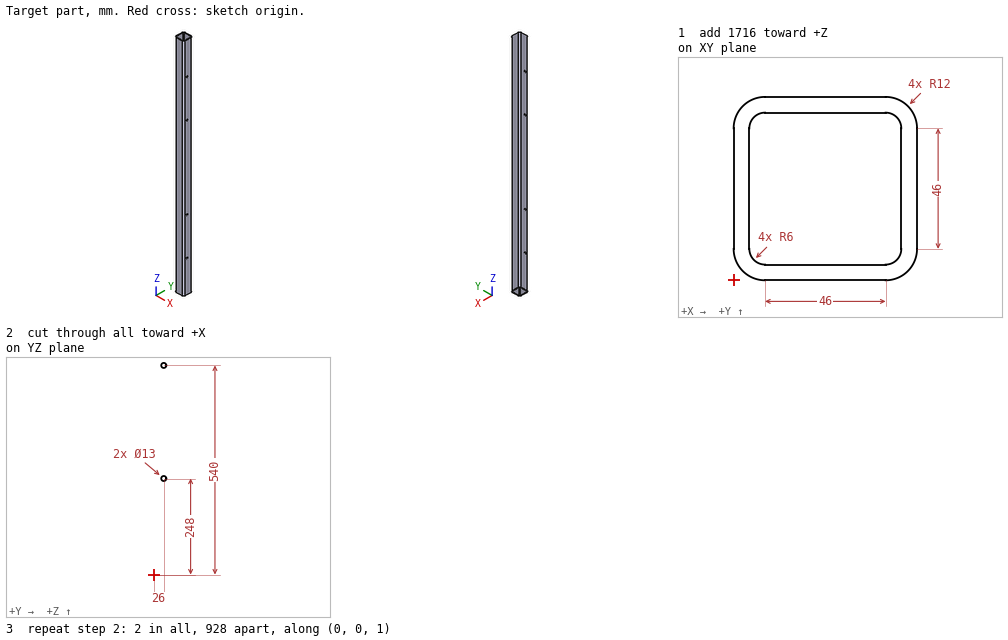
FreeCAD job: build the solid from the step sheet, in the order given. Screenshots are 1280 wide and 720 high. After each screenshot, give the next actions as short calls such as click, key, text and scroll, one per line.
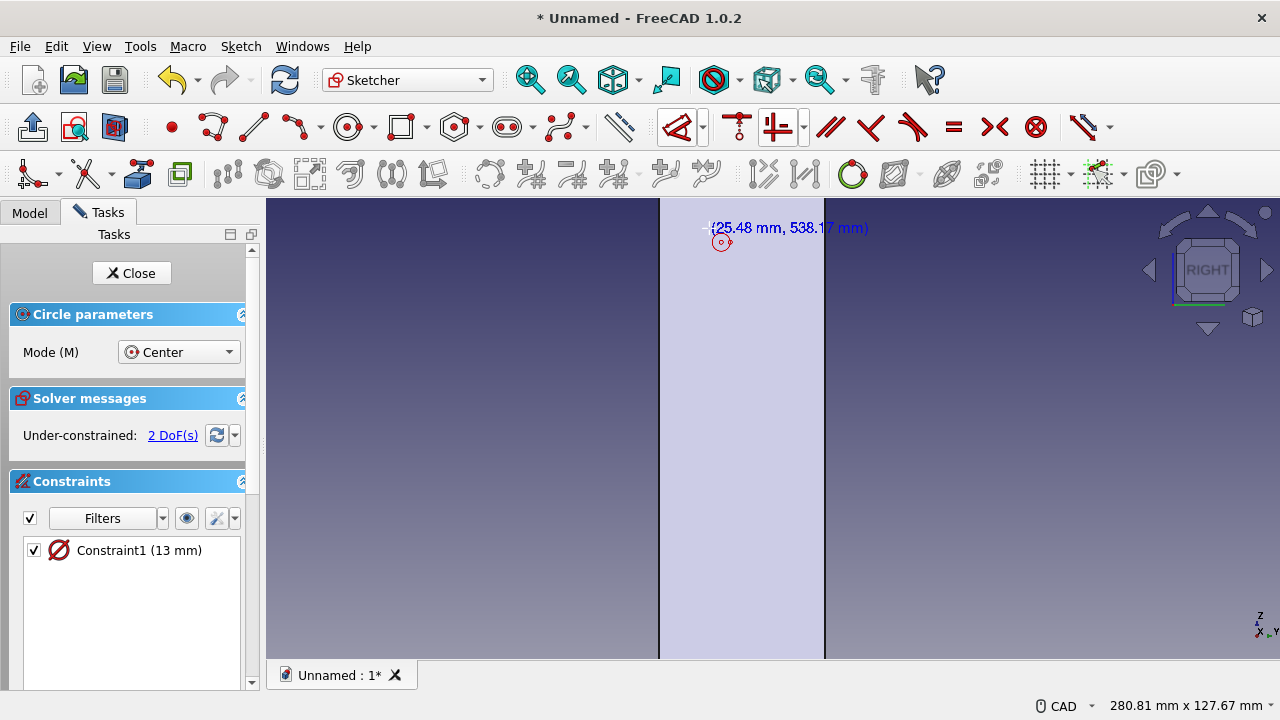
scroll(709, 309, down, 10)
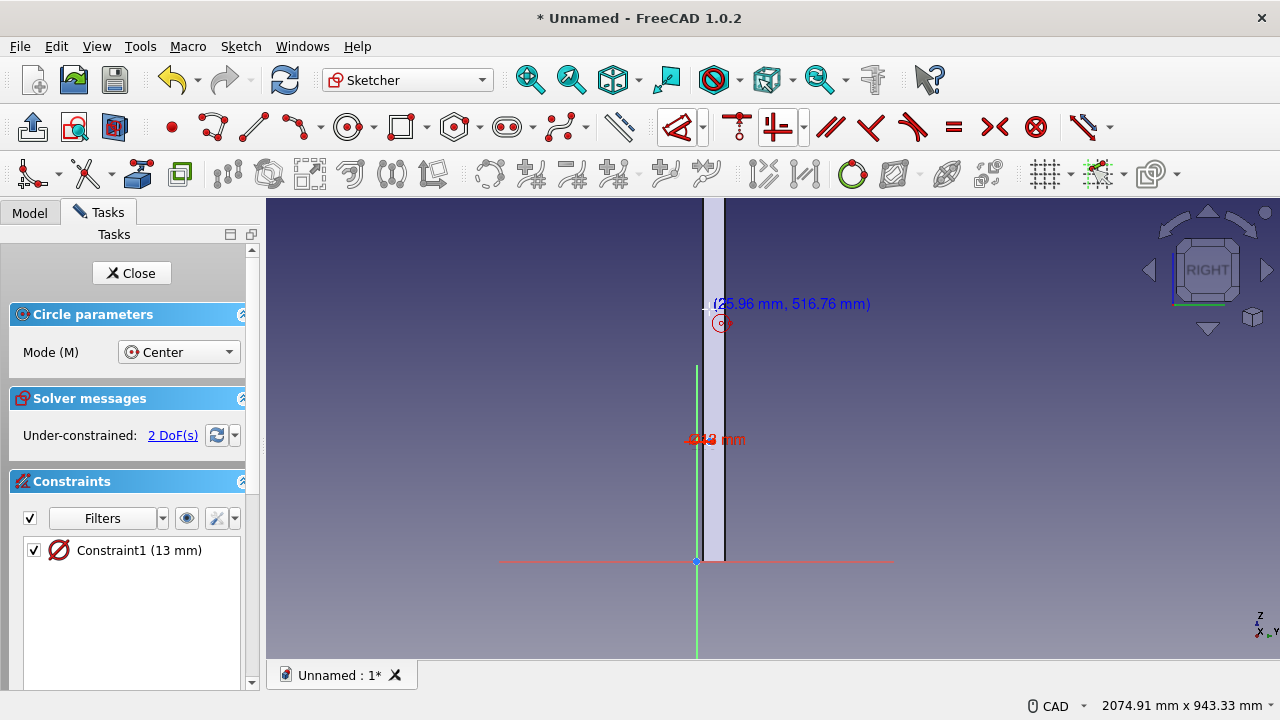
scroll(709, 298, up, 2)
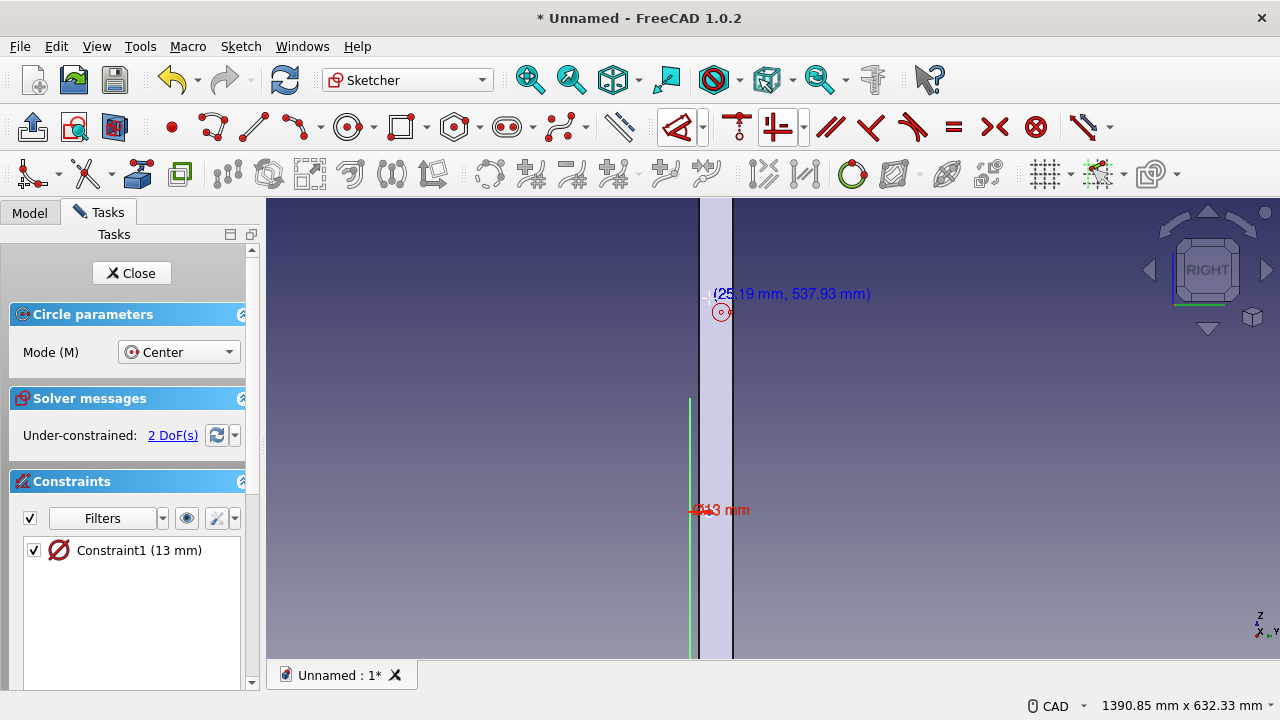
click(709, 298)
move(713, 295)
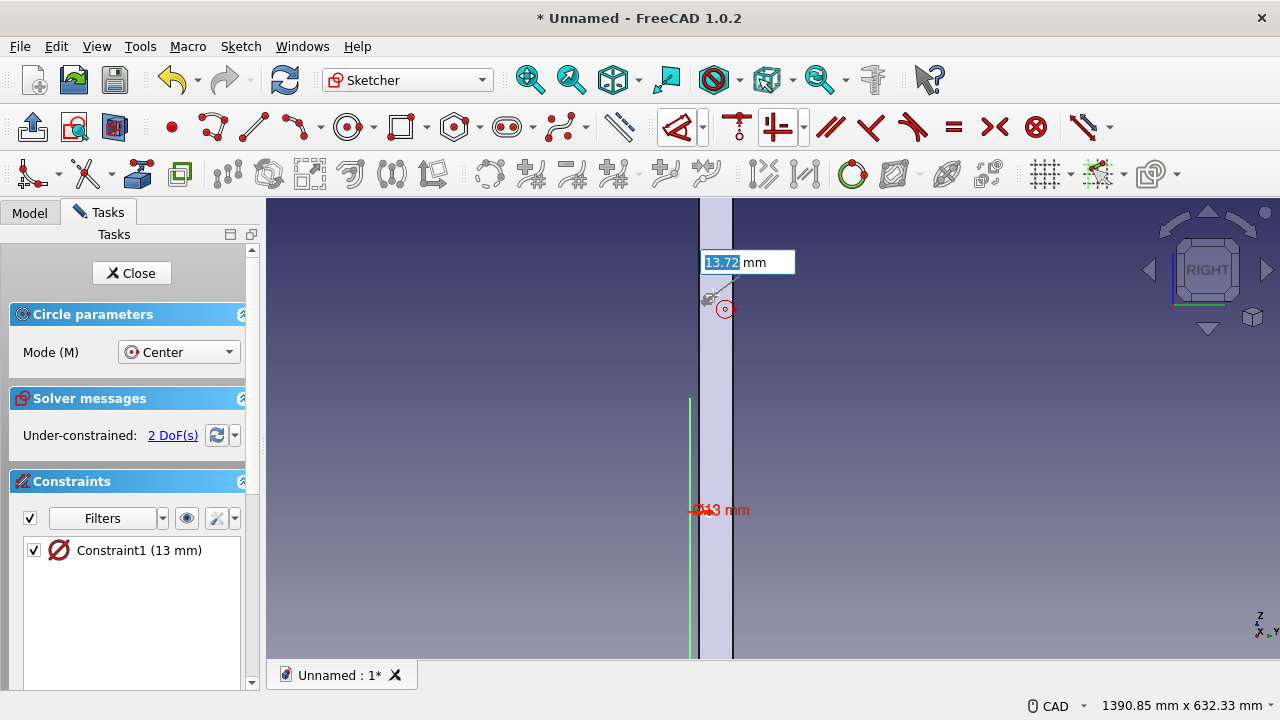
text(13)
key(Return)
key(Escape)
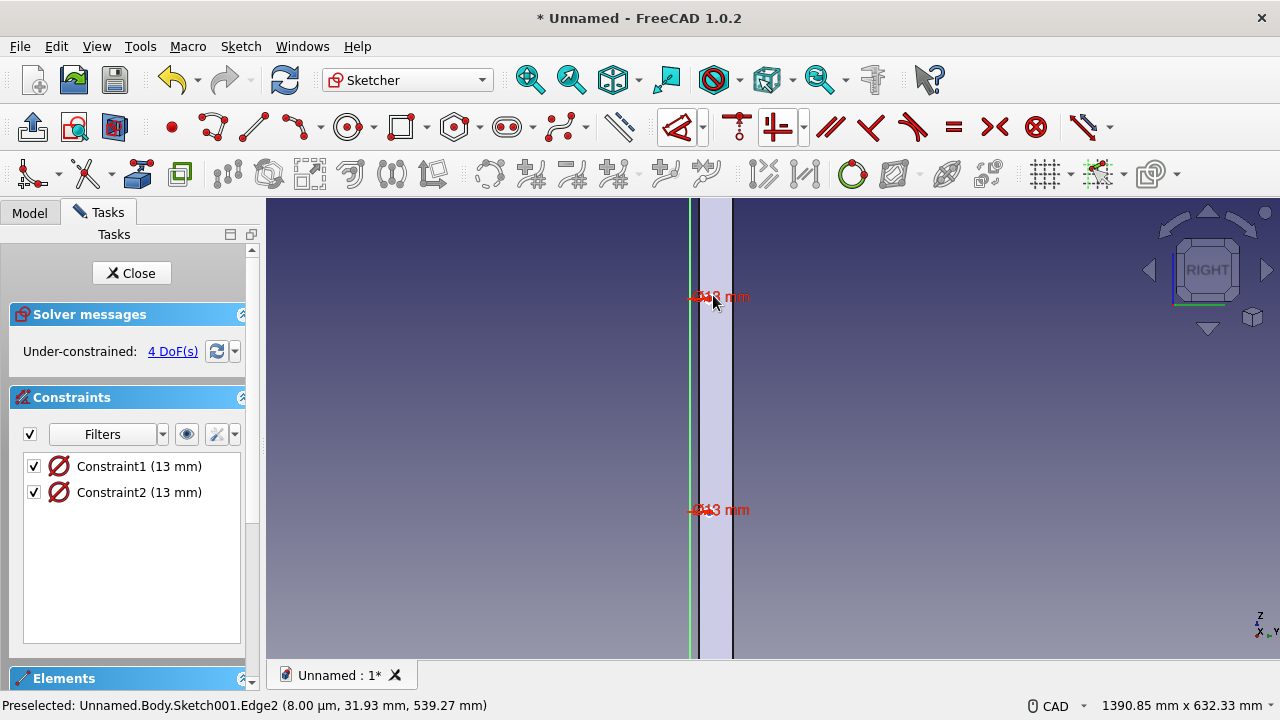
click(709, 512)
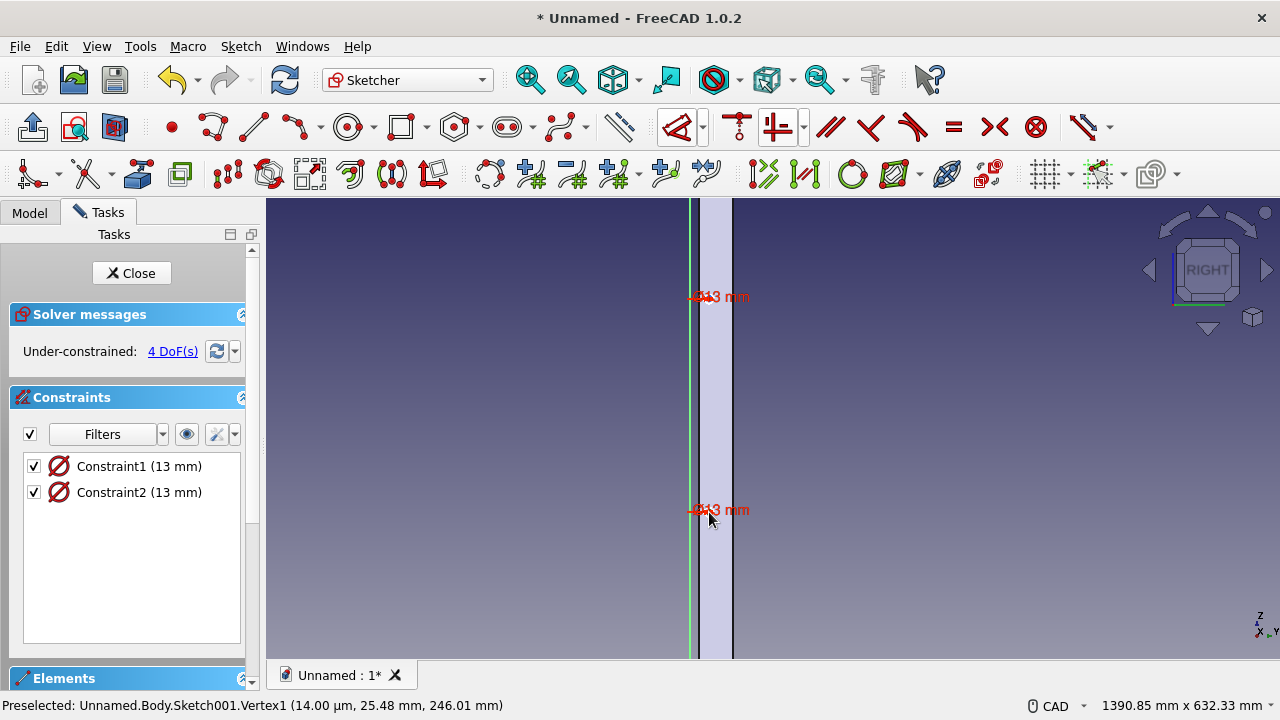
click(709, 299)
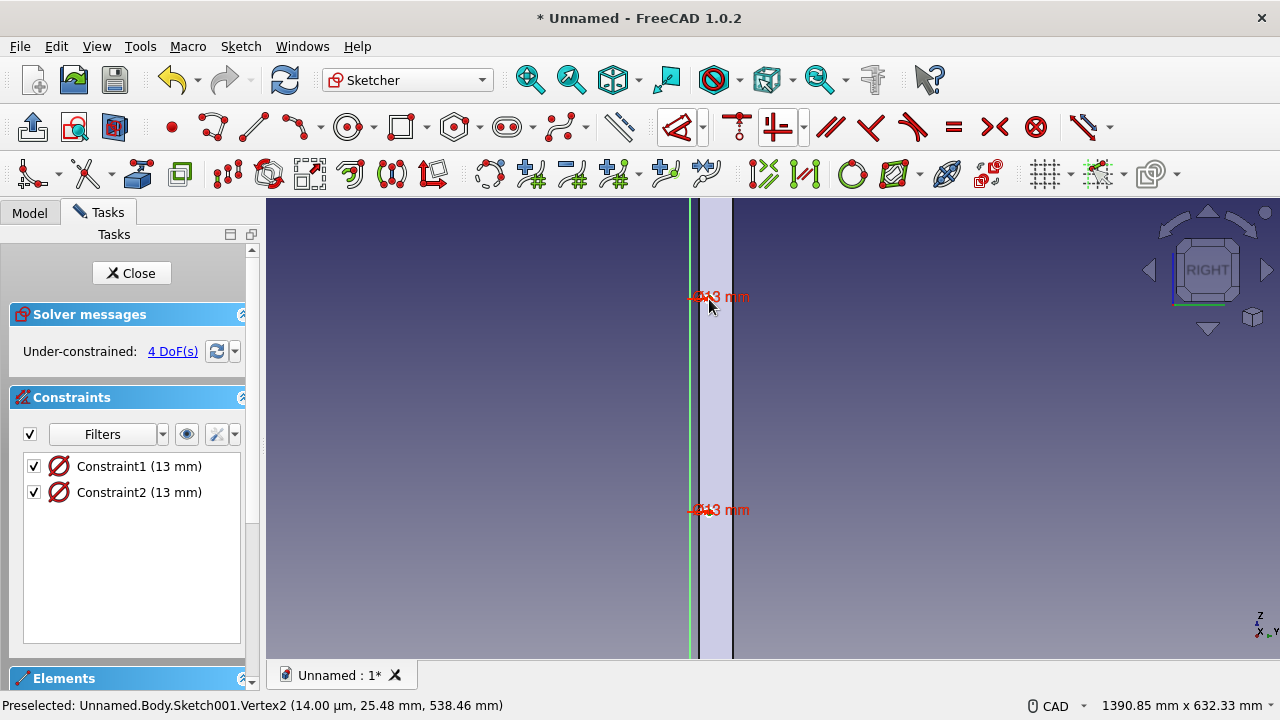
click(804, 128)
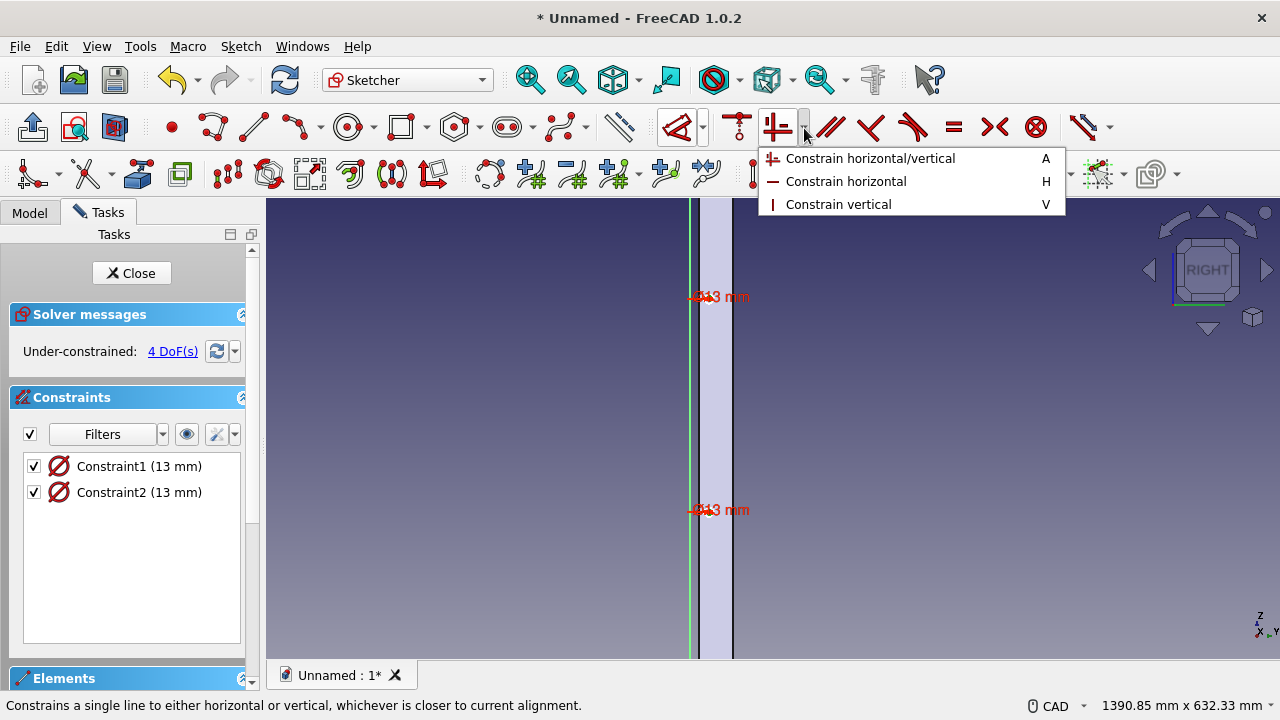
click(912, 204)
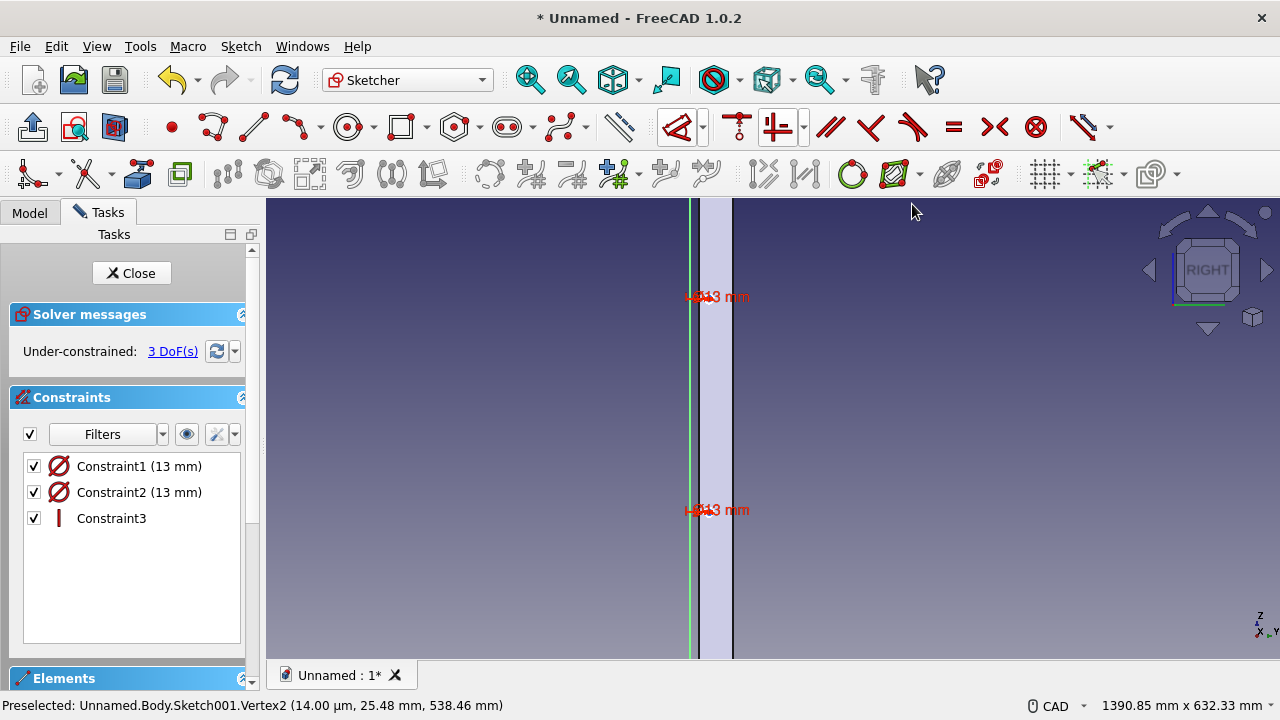
scroll(709, 512, up, 4)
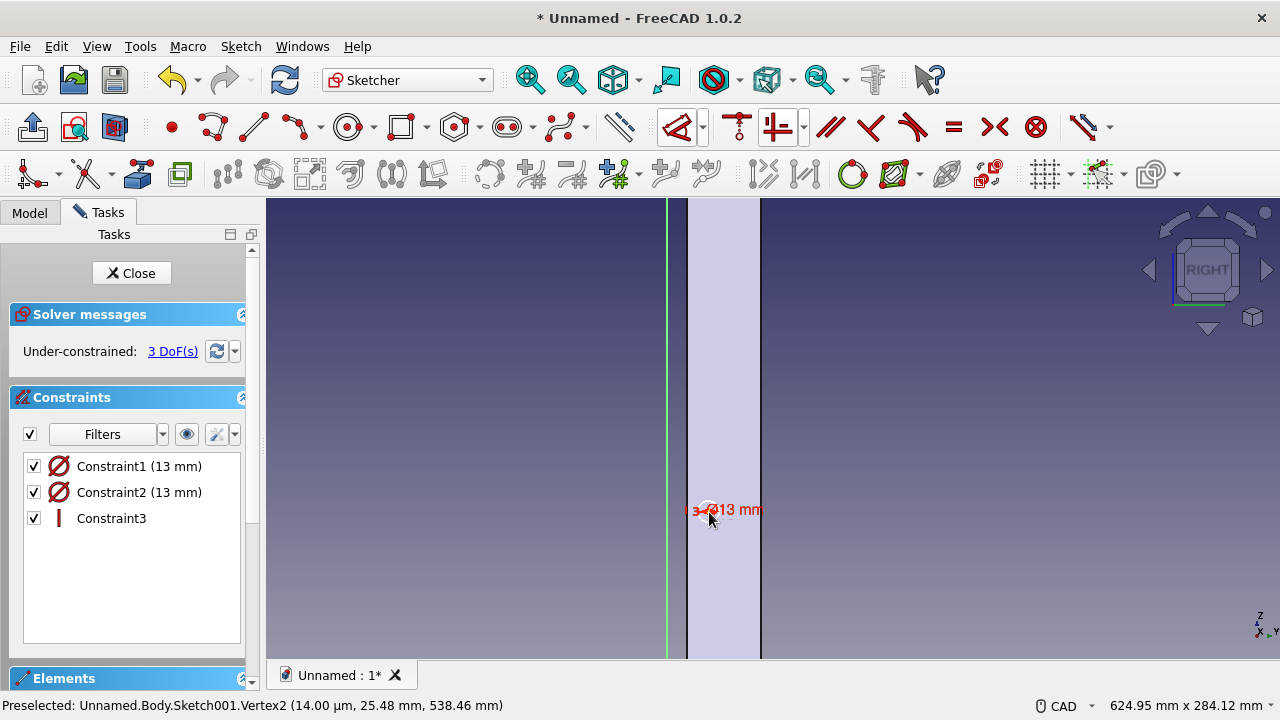
click(708, 512)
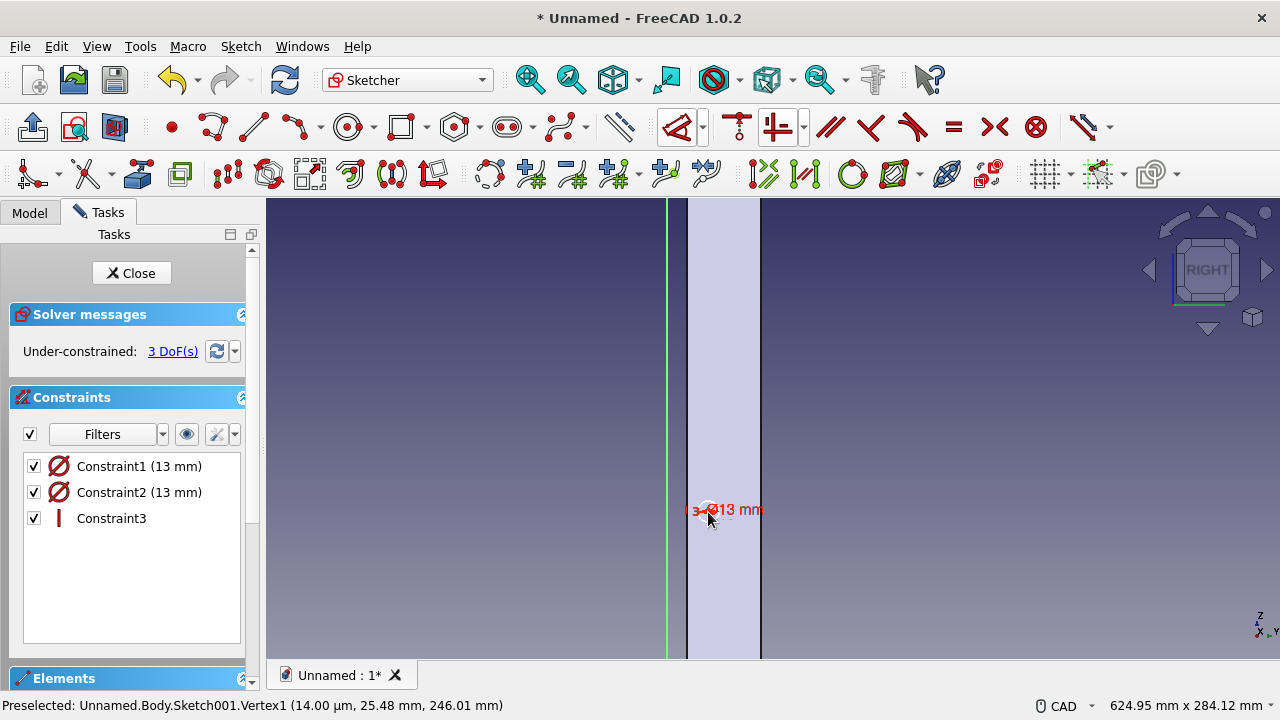
key(l)